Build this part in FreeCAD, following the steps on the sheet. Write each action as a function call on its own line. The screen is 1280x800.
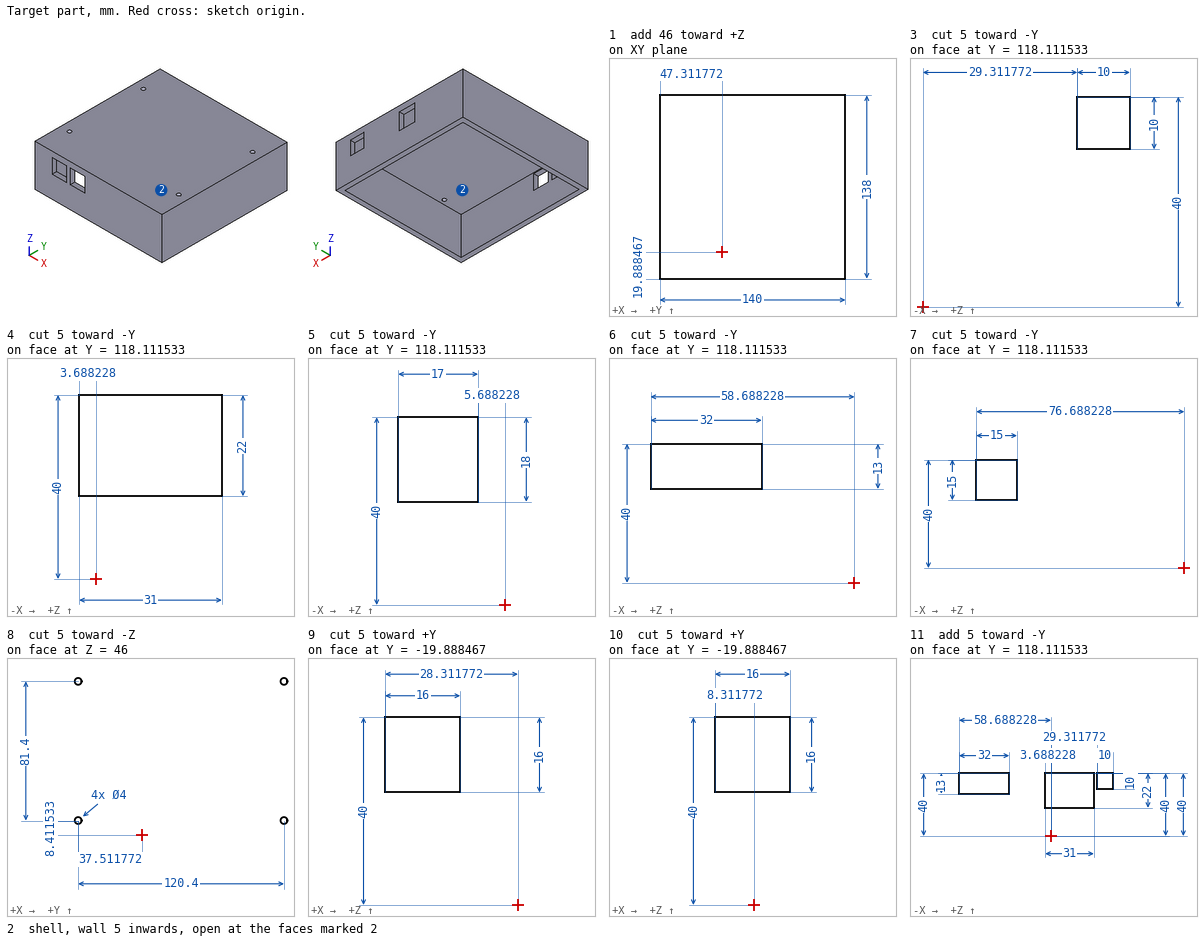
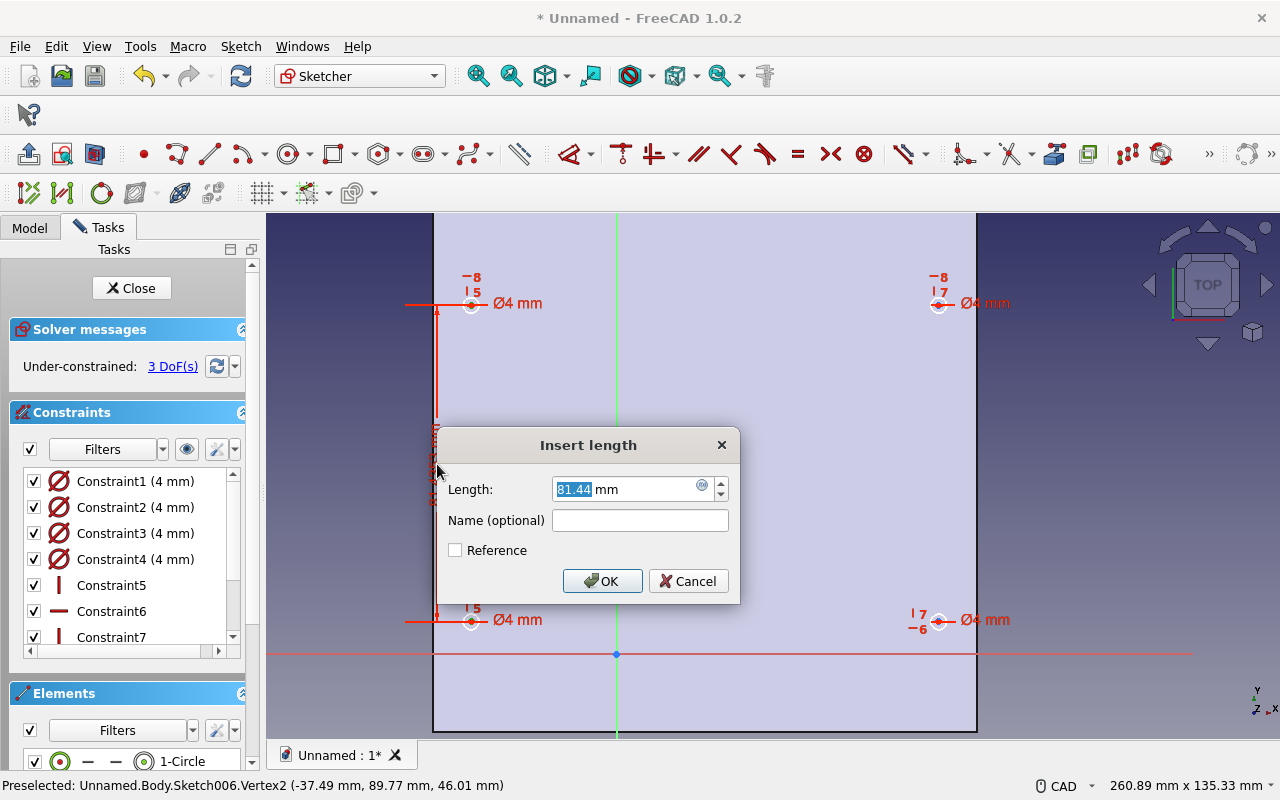
text(81.4)
key(Return)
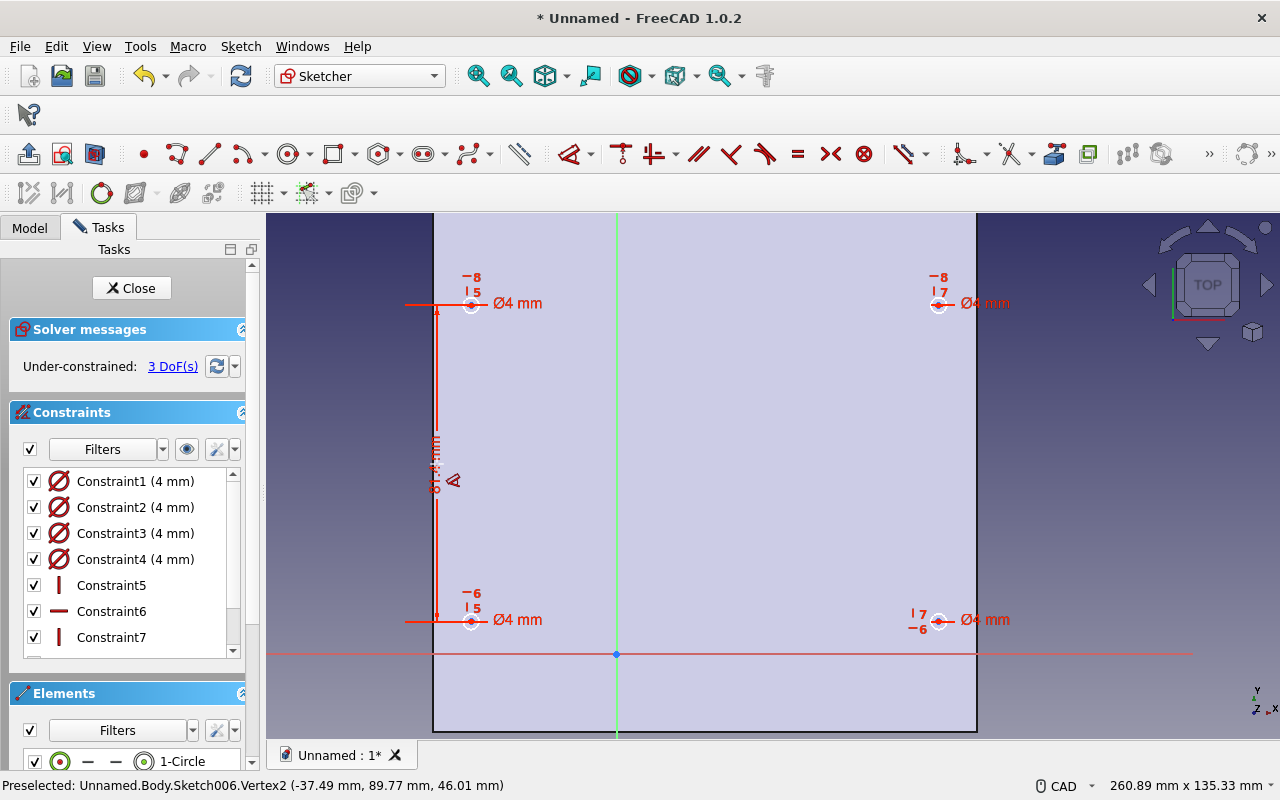
click(471, 622)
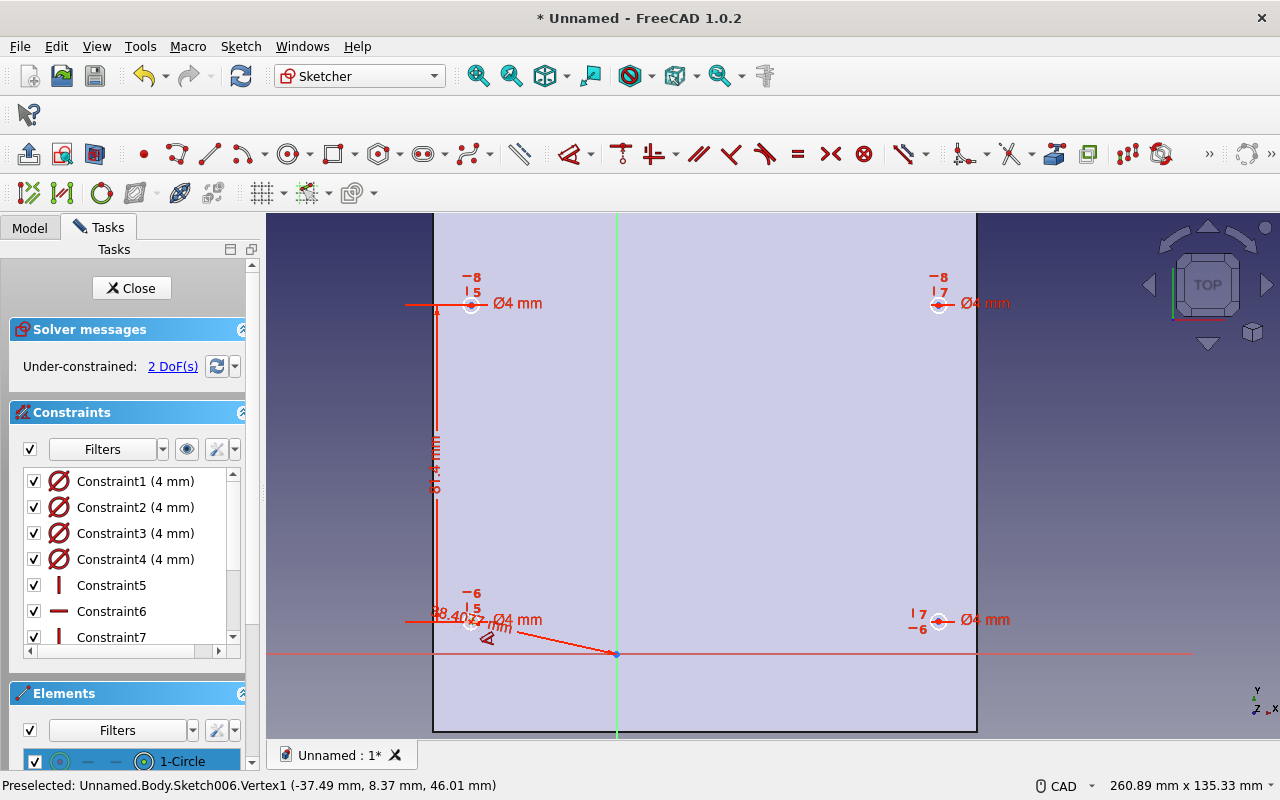
click(939, 622)
click(705, 588)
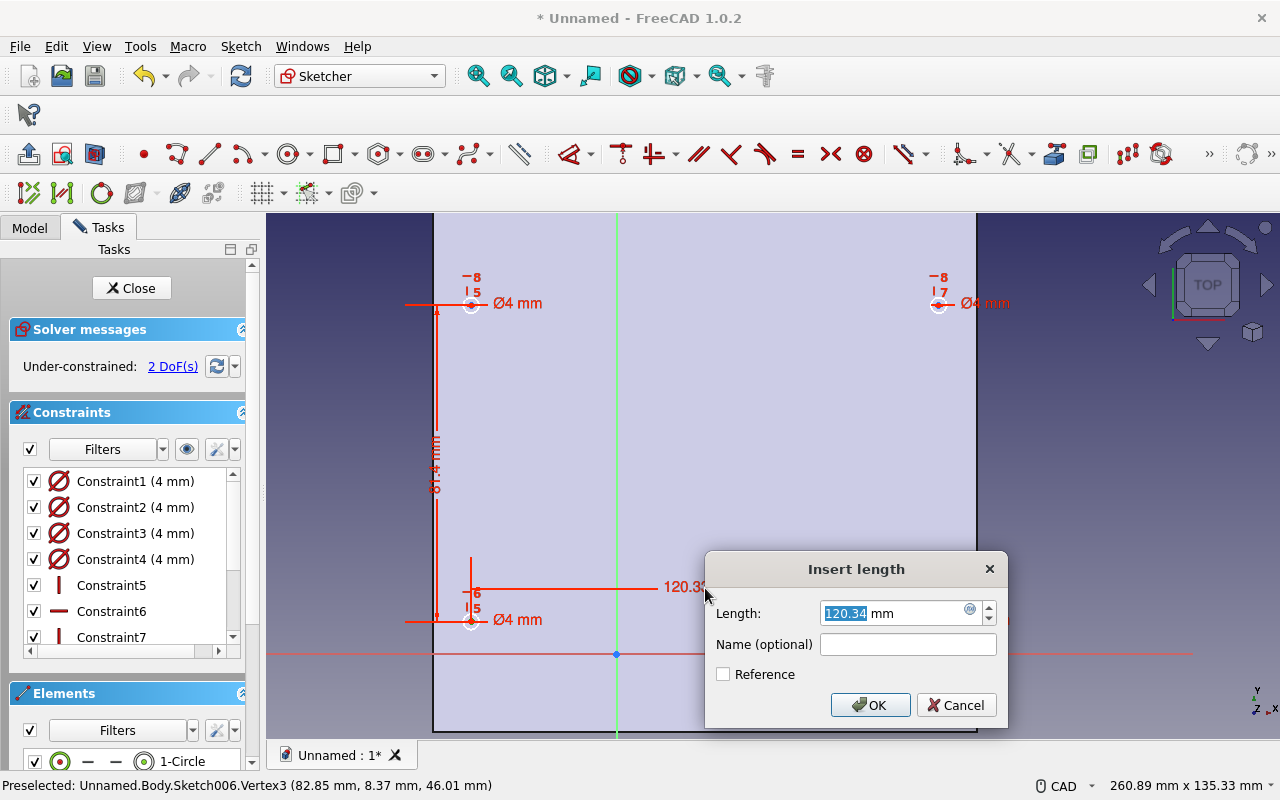
text(120.4)
key(Return)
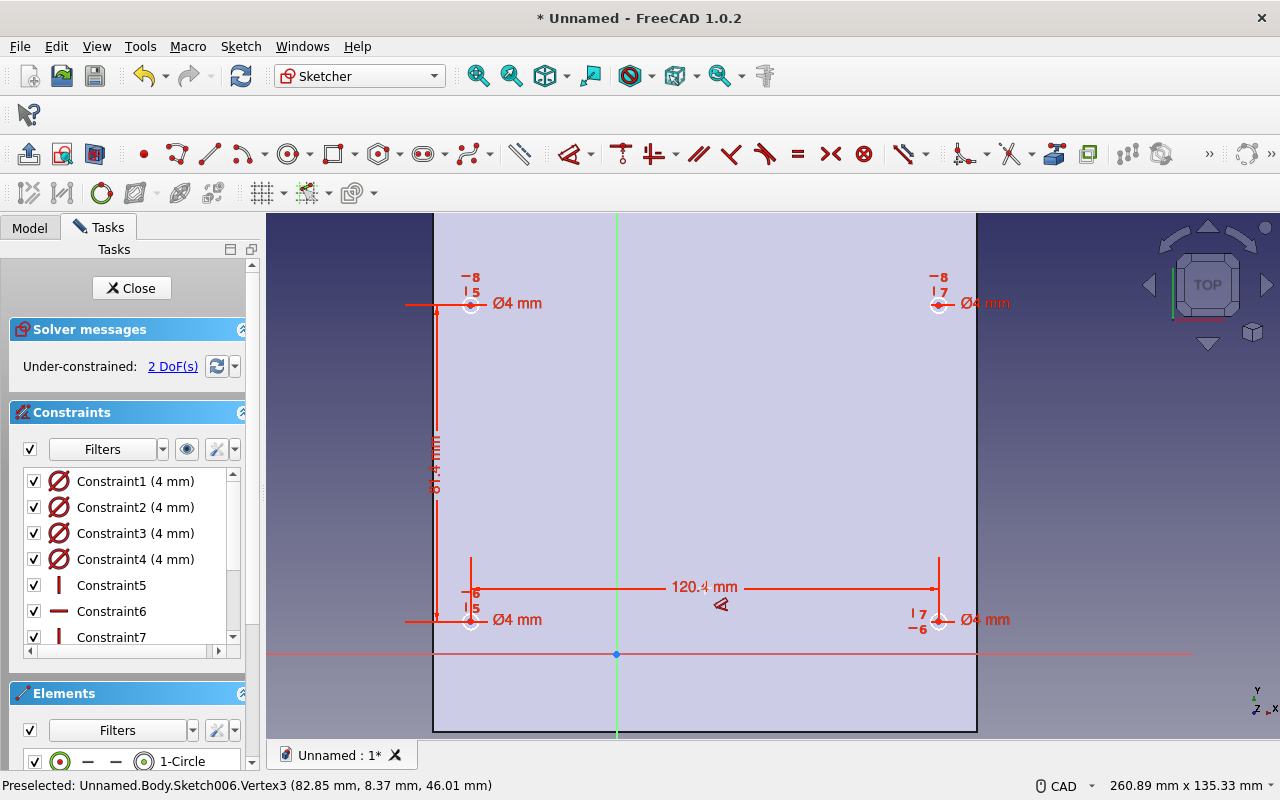
click(471, 622)
click(437, 638)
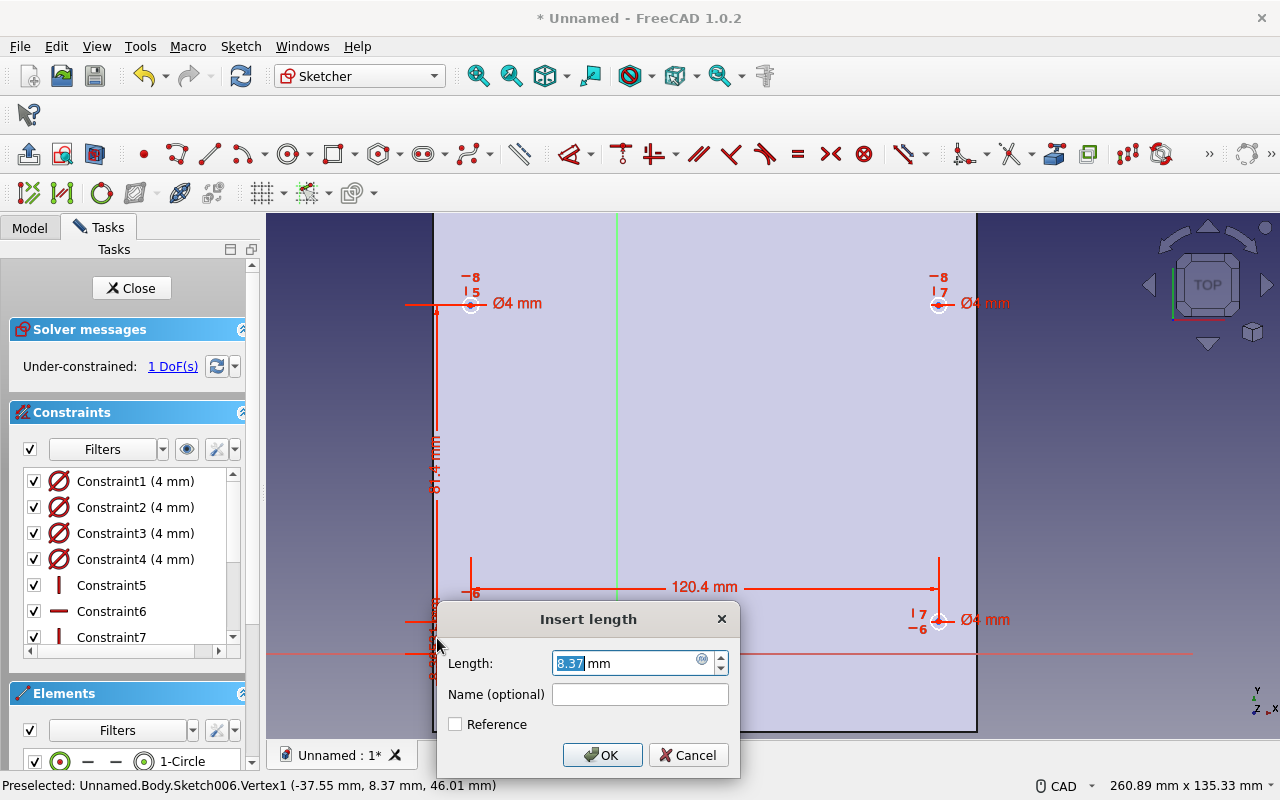
text(8.411533)
key(Return)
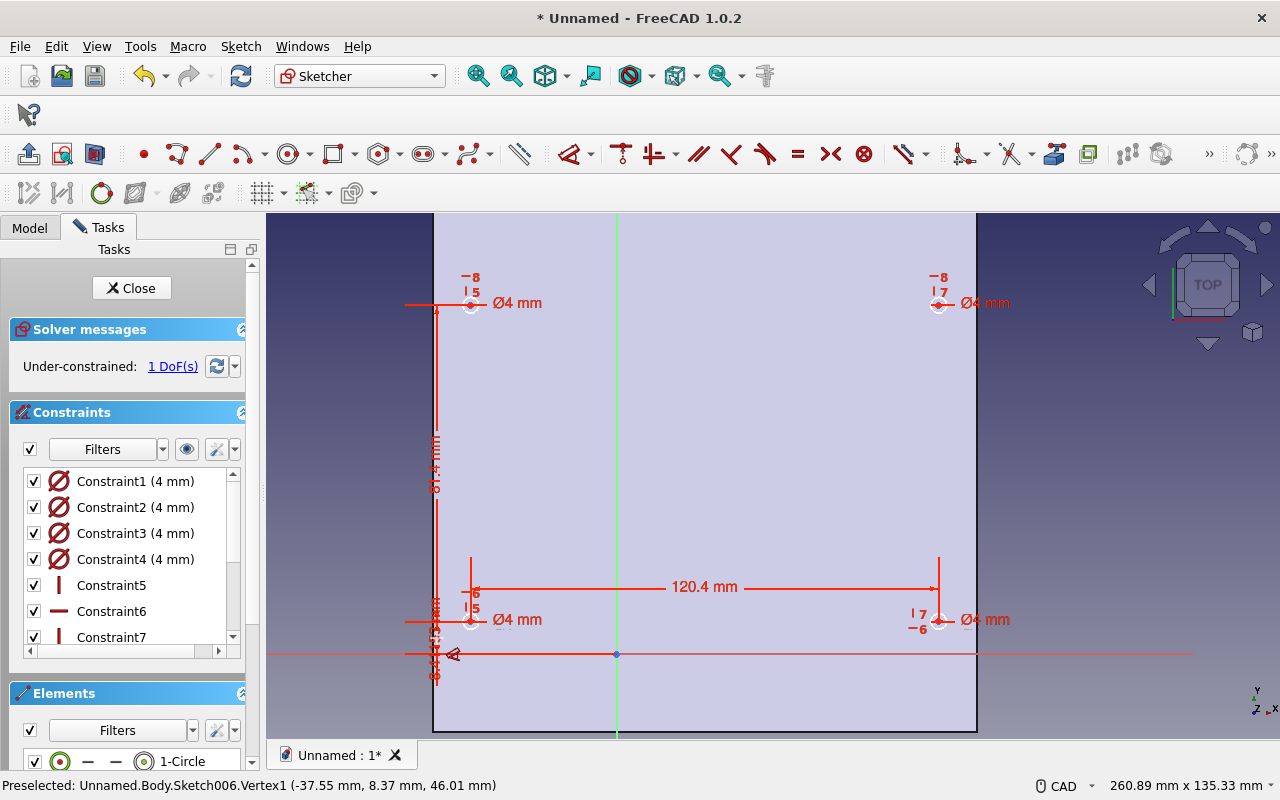
click(471, 622)
click(544, 688)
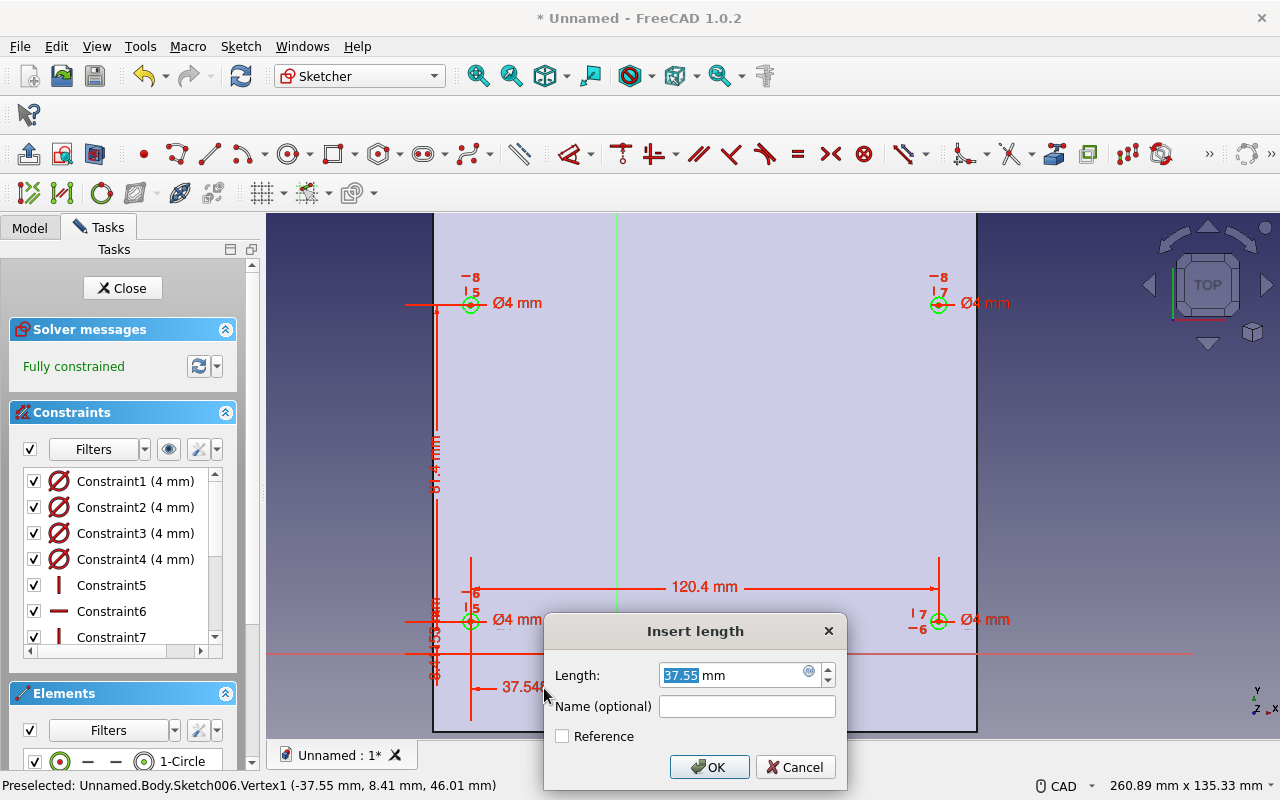
text(37.511772)
key(Return)
key(Escape)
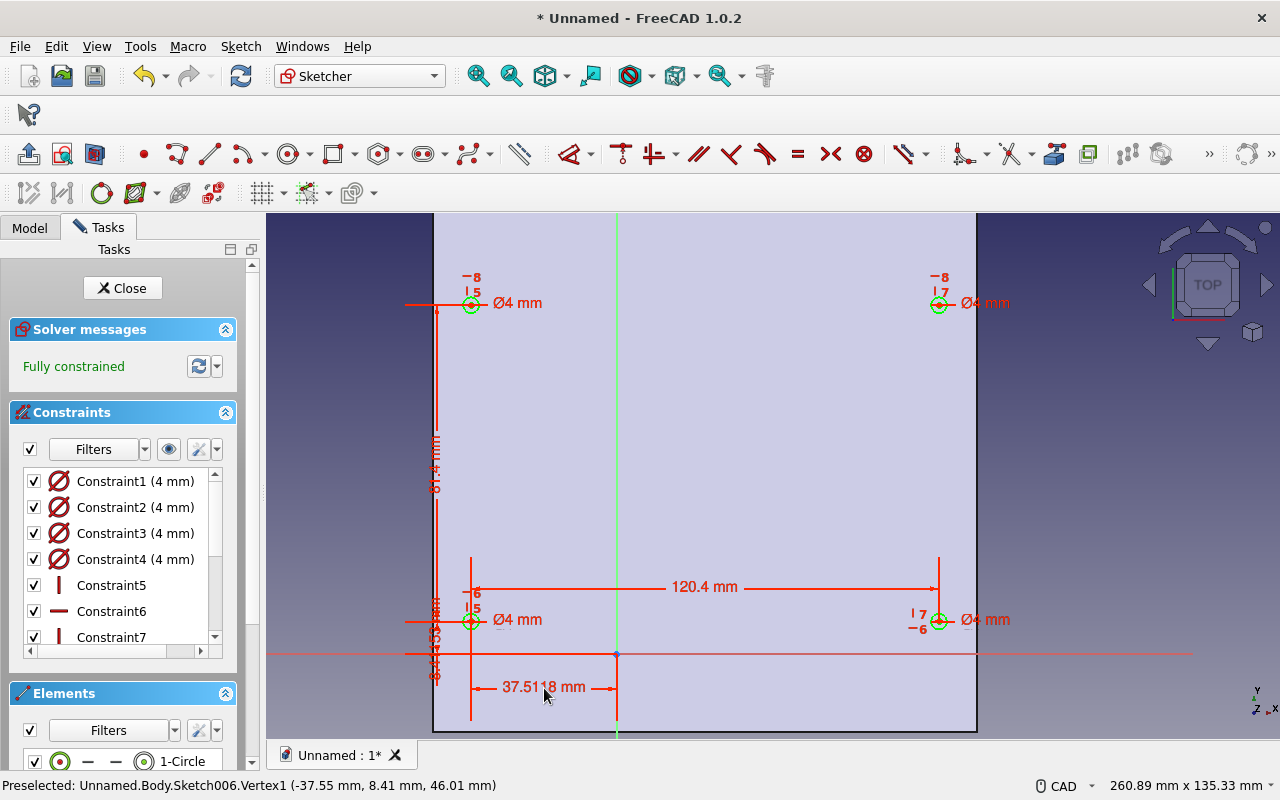
click(123, 288)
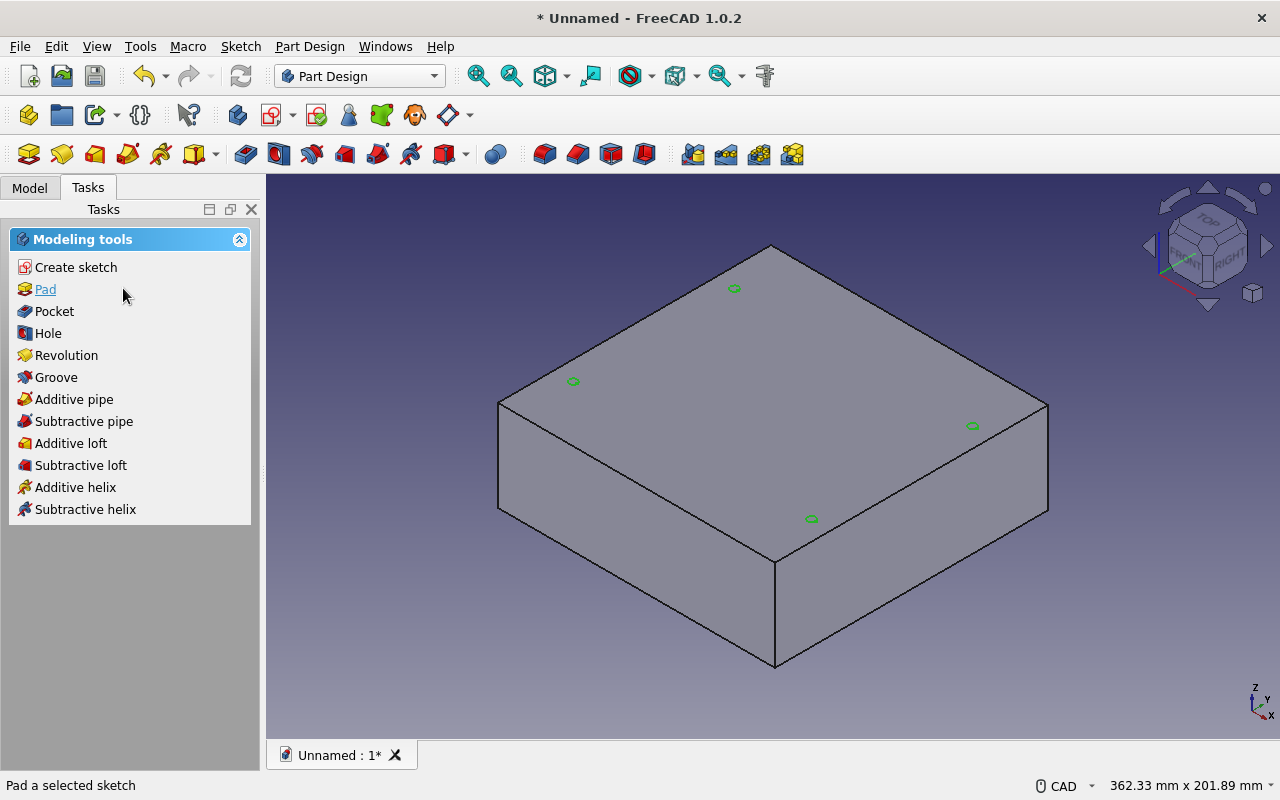
click(246, 154)